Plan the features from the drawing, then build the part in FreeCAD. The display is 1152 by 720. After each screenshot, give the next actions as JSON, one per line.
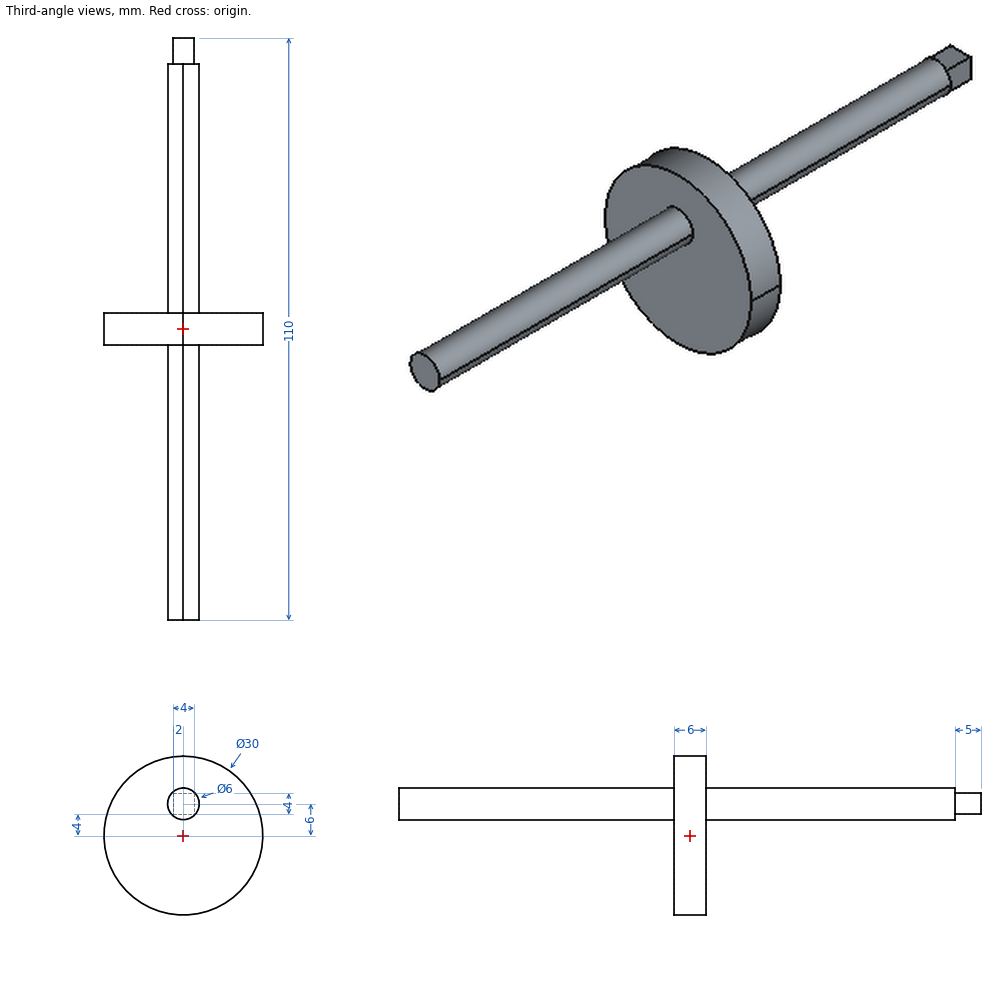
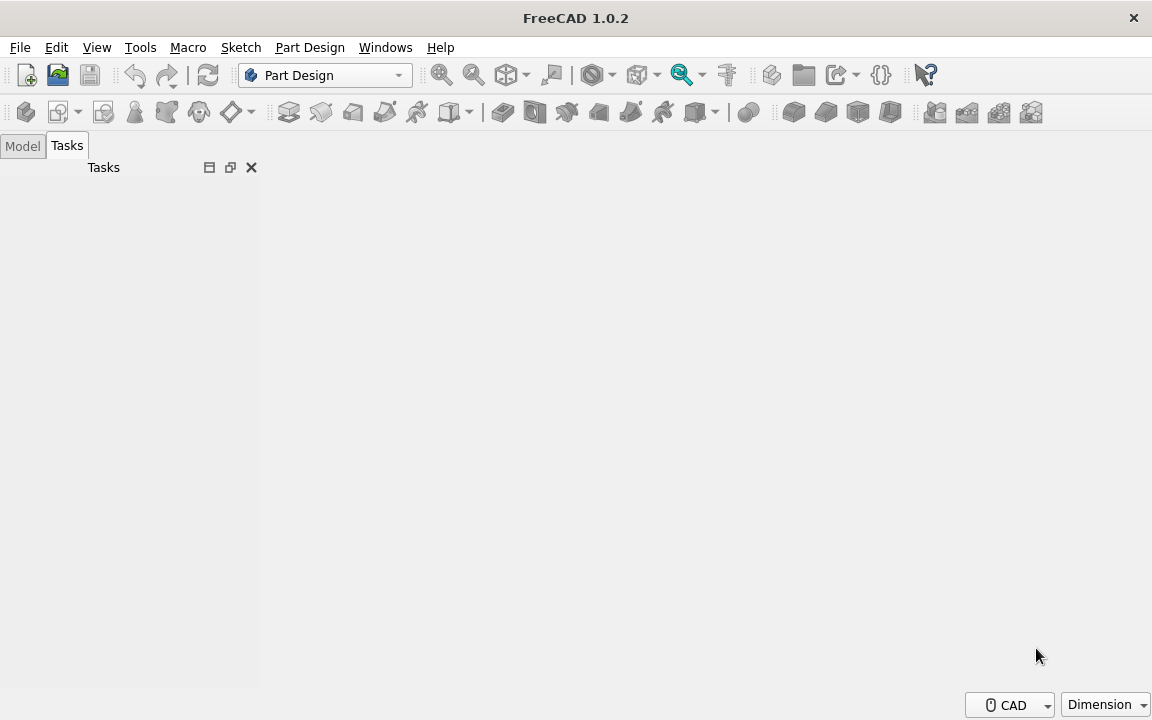
{"action": "key", "text": "ctrl+n"}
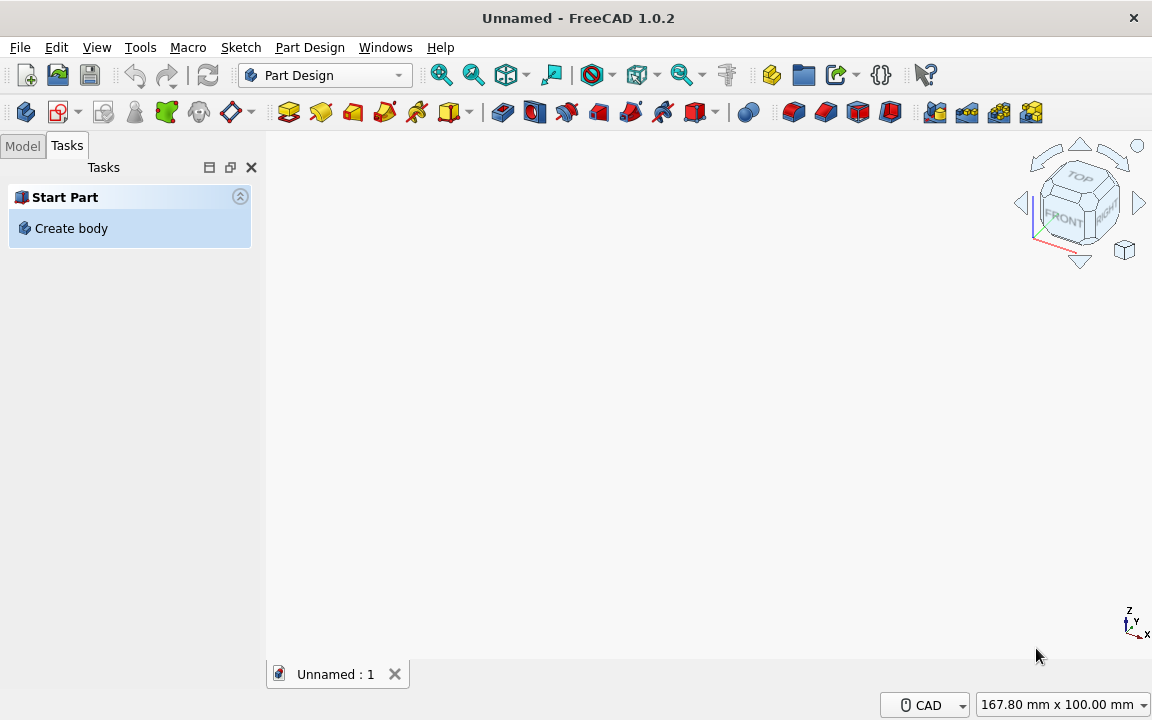
{"action": "left_click", "coordinate": [58, 112]}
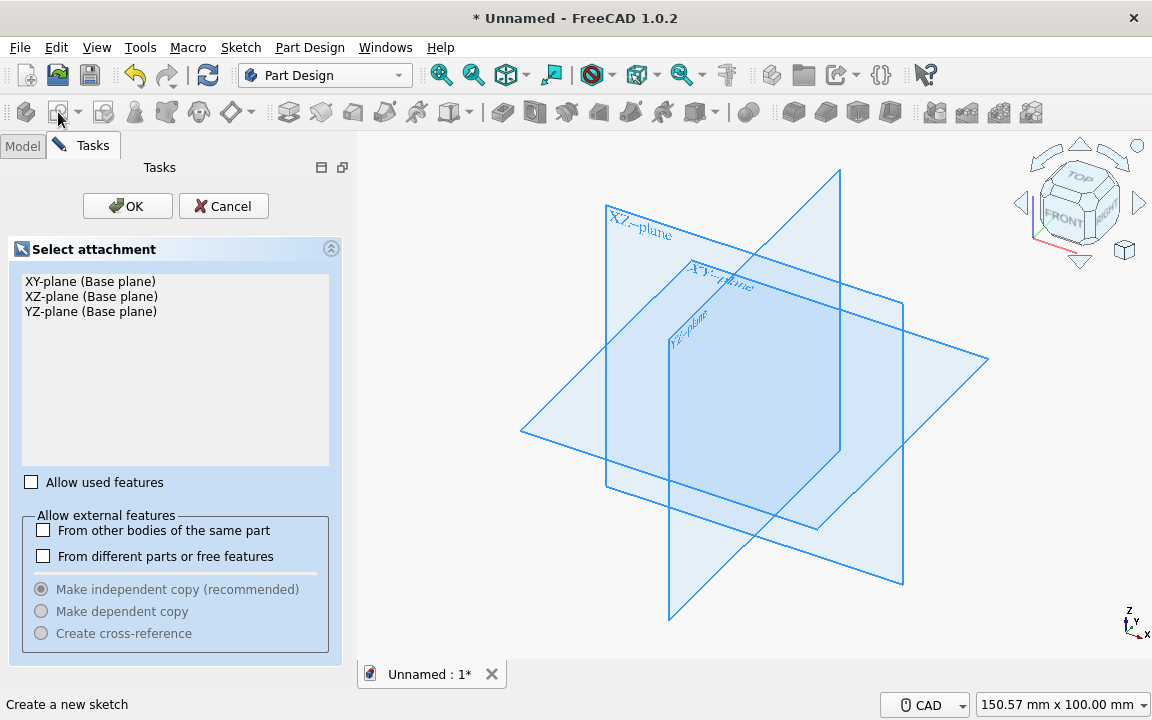
{"action": "left_click", "coordinate": [82, 296]}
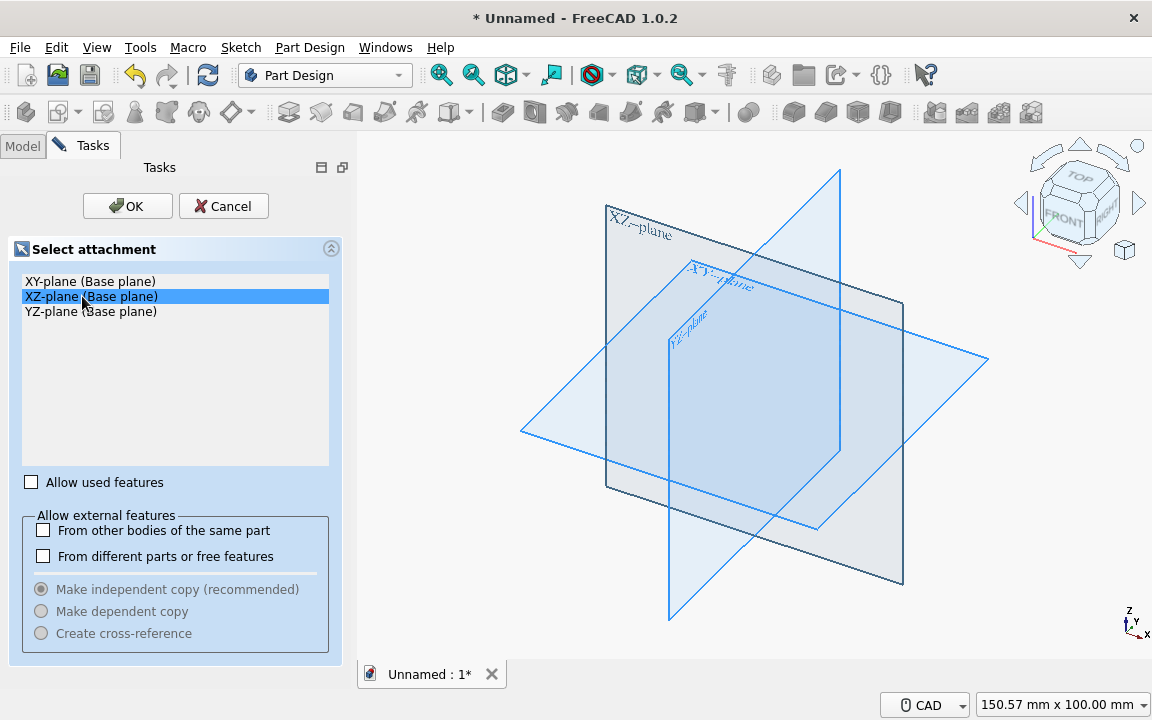
{"action": "left_click", "coordinate": [128, 206]}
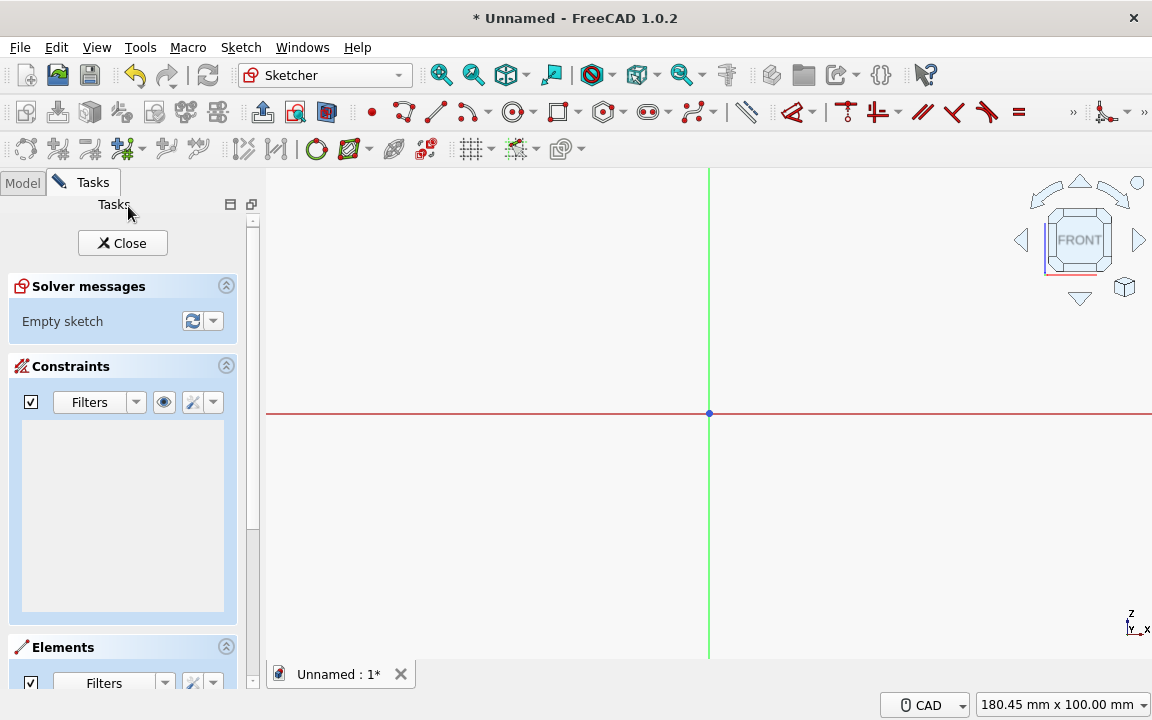
{"action": "scroll", "coordinate": [765, 413], "scroll_direction": "up", "scroll_amount": 4}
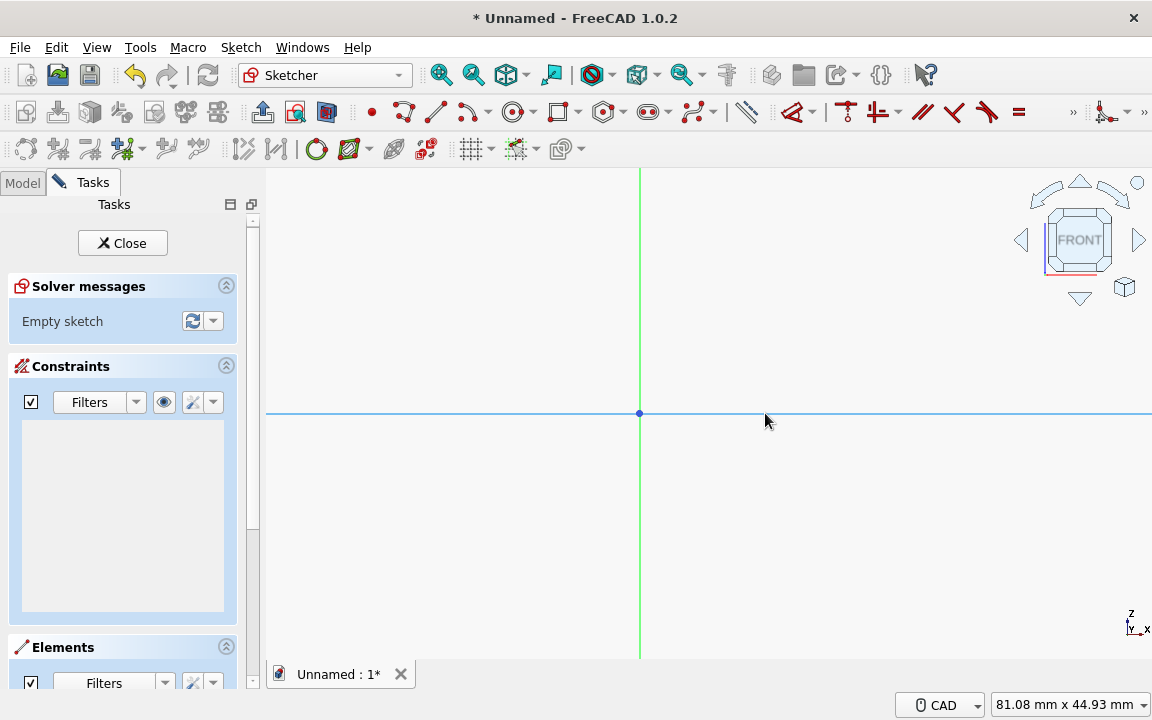
{"action": "left_click", "coordinate": [514, 112]}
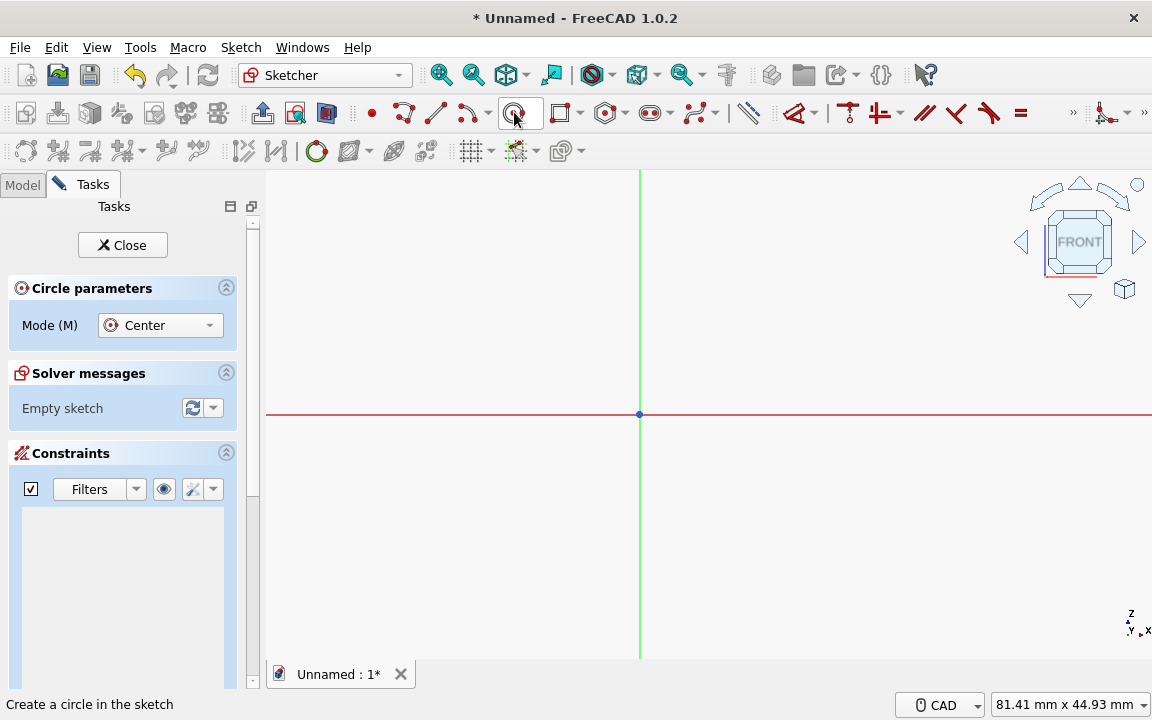
{"action": "left_click", "coordinate": [640, 414]}
{"action": "mouse_move", "coordinate": [755, 299]}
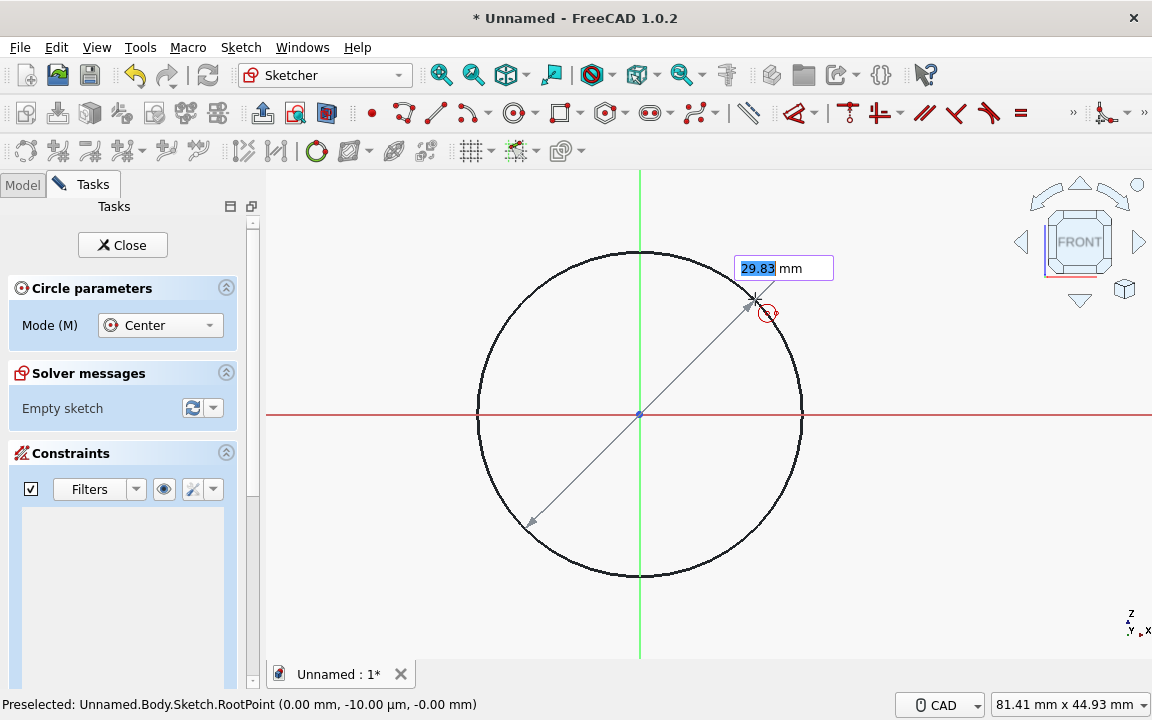
{"action": "type", "text": "30"}
{"action": "key", "text": "Return"}
{"action": "key", "text": "Escape"}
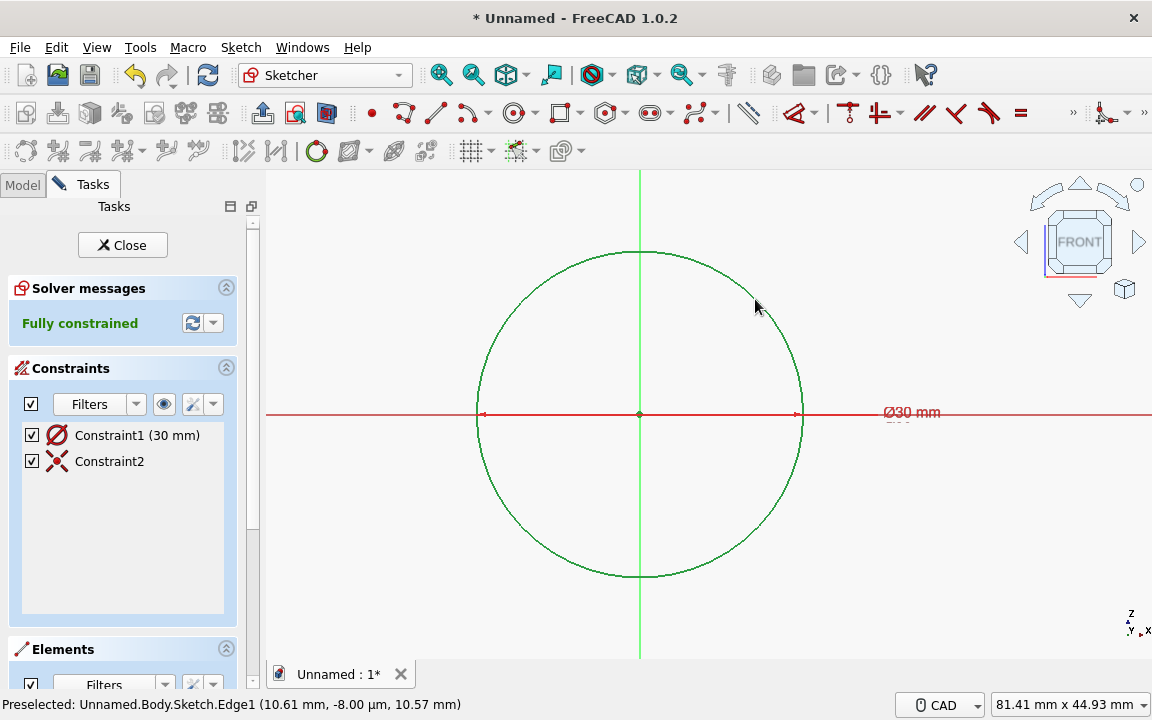
{"action": "left_click", "coordinate": [123, 245]}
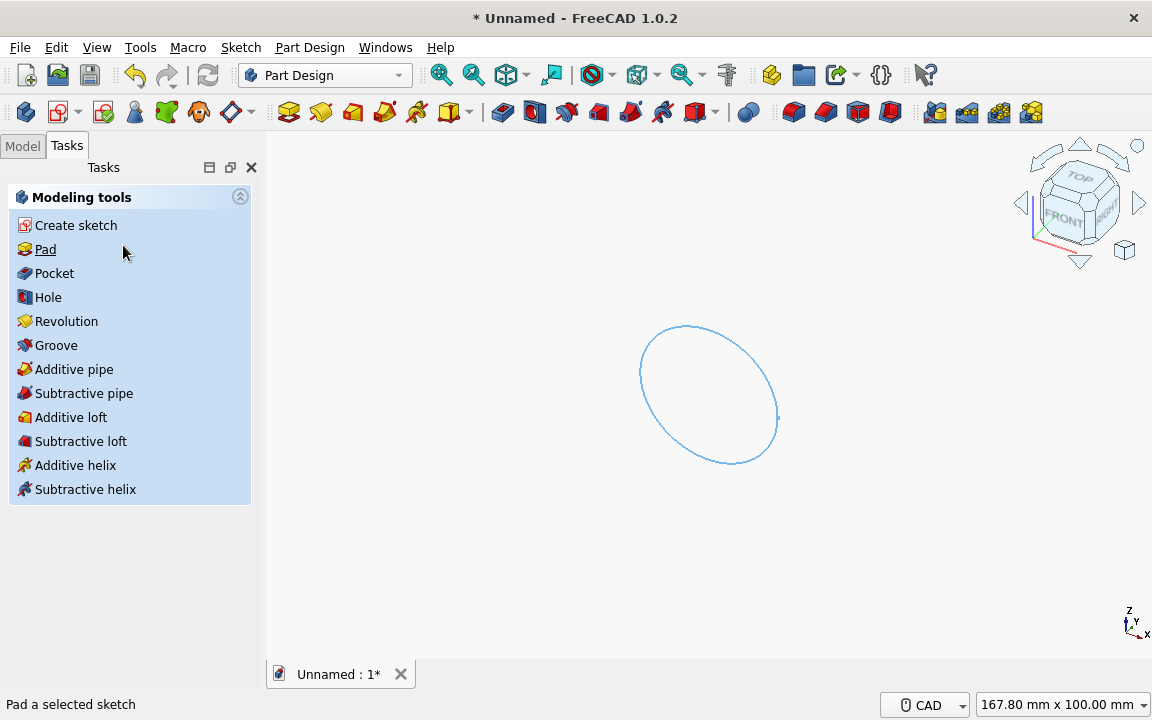
{"action": "left_click", "coordinate": [290, 112]}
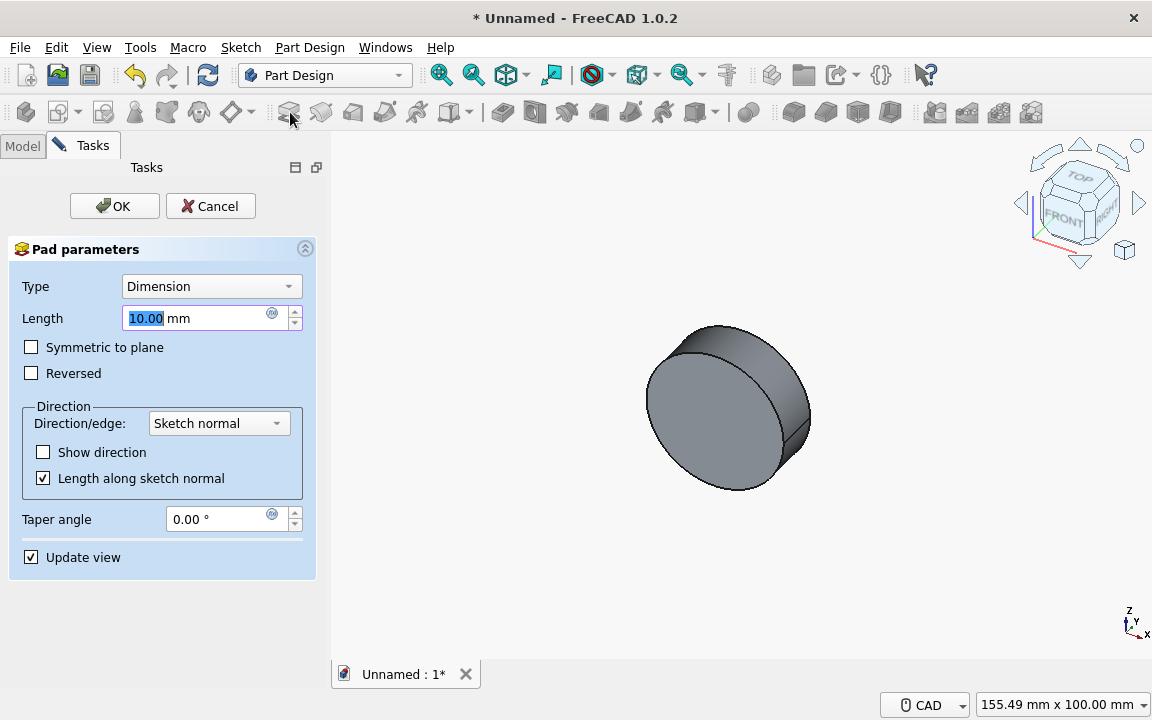
{"action": "type", "text": "6"}
{"action": "key", "text": "Tab"}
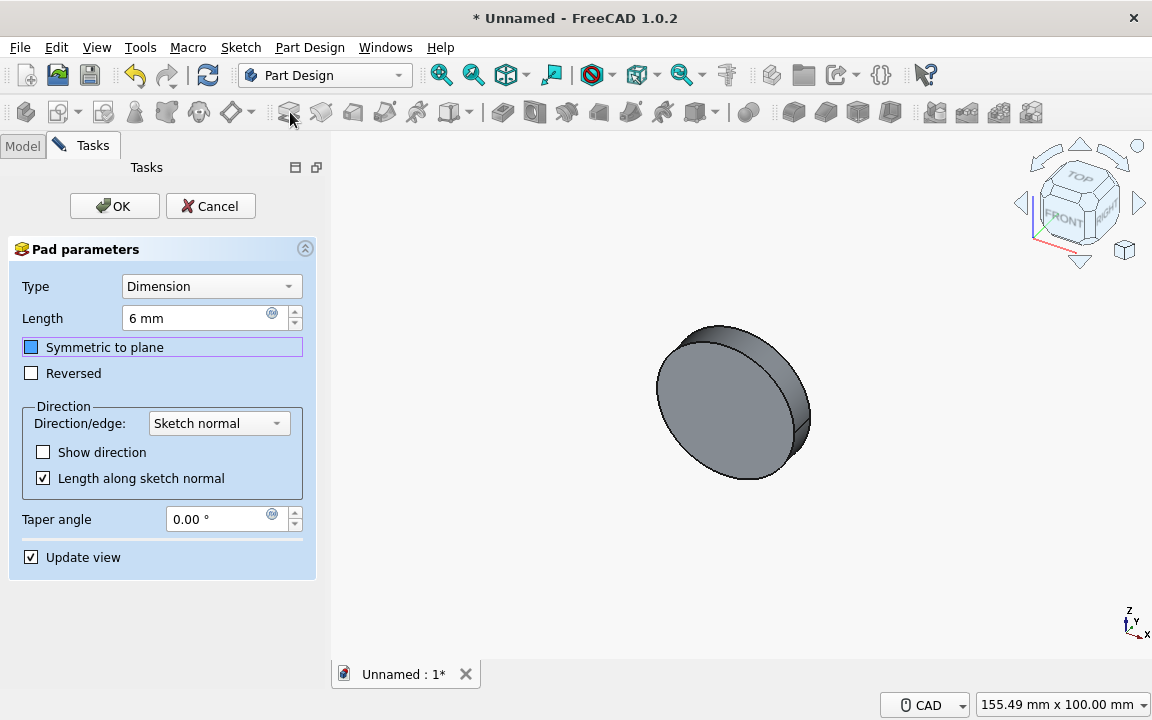
{"action": "left_click", "coordinate": [30, 347]}